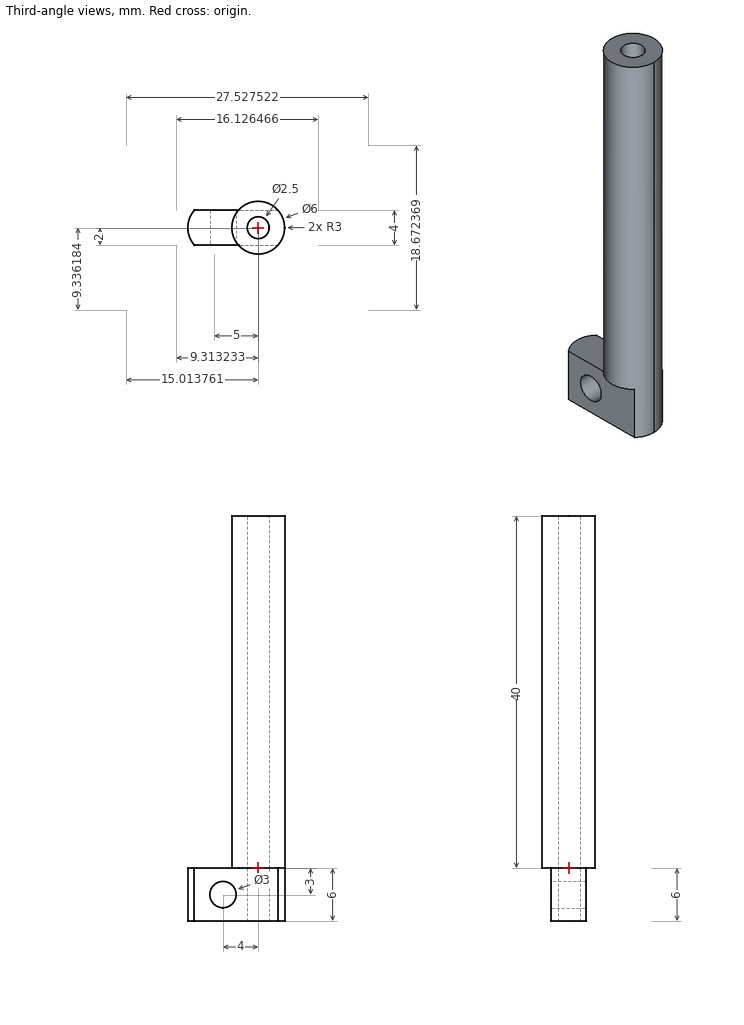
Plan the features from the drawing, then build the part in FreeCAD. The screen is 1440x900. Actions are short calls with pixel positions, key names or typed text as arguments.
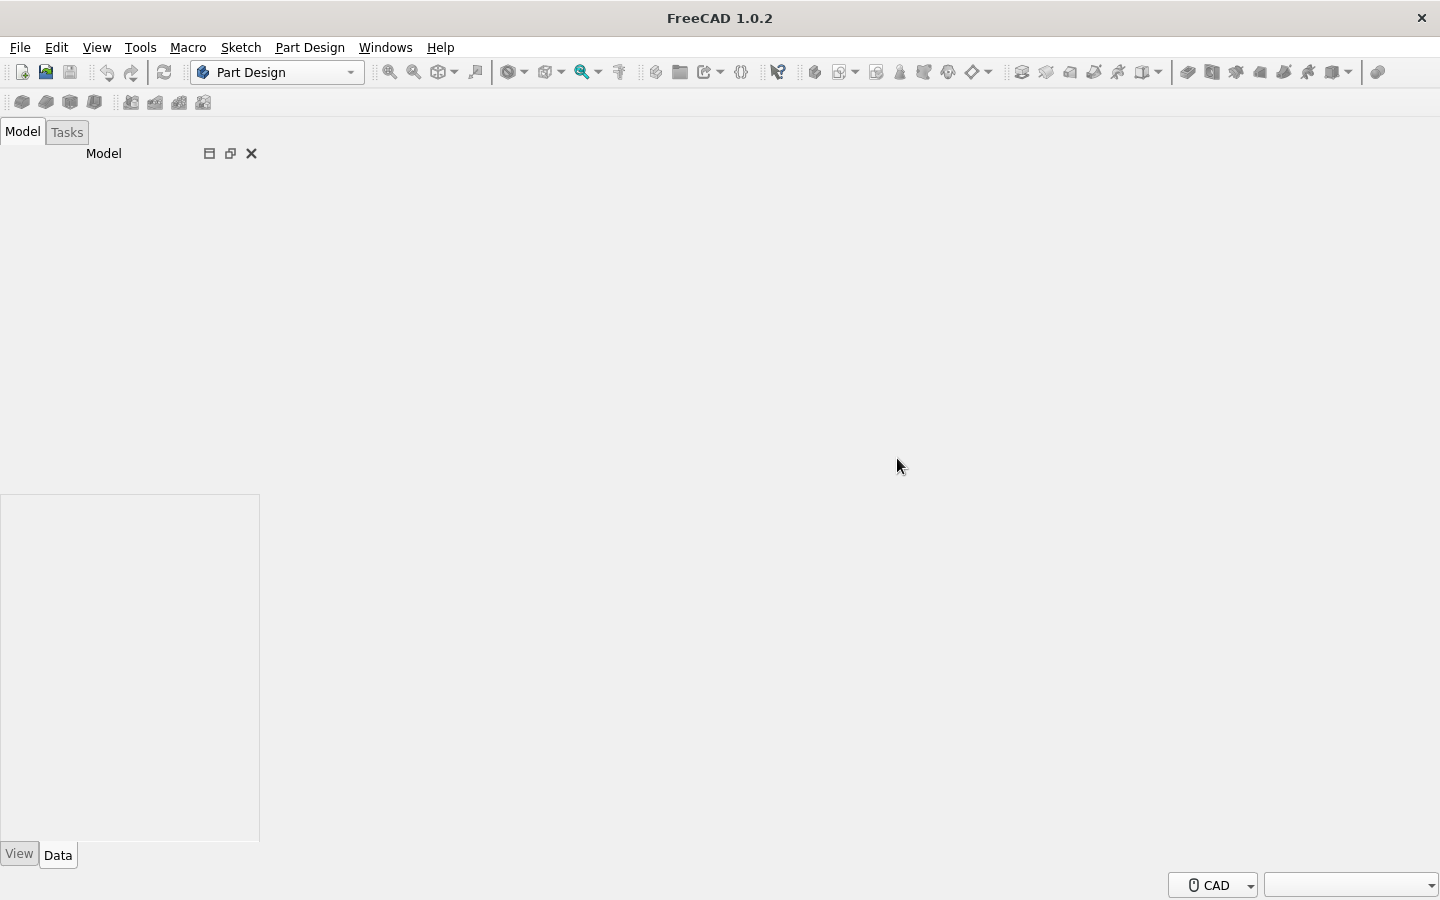
key(ctrl+n)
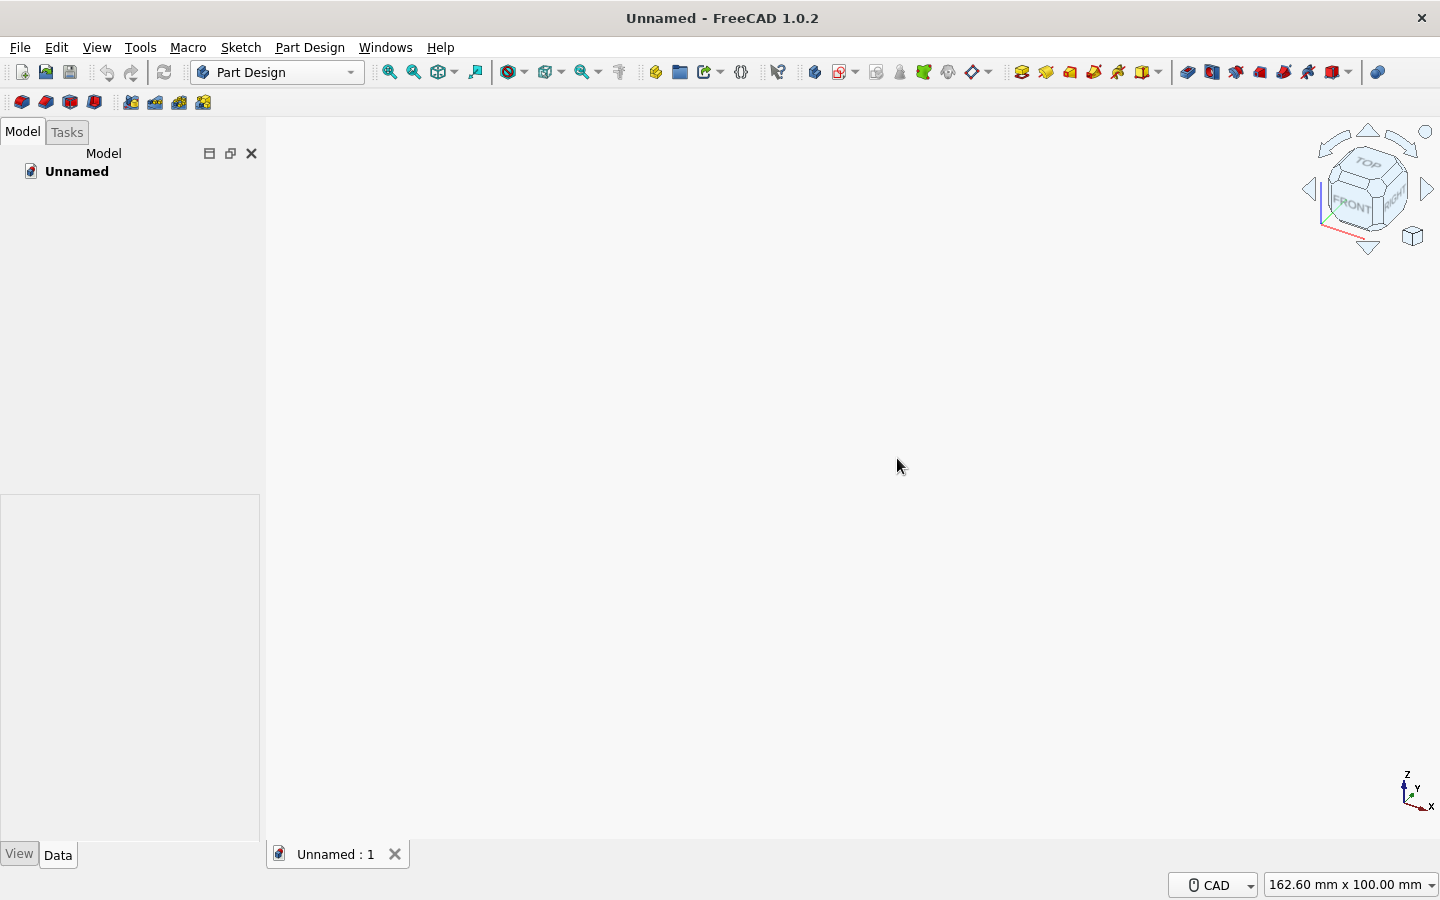
click(840, 72)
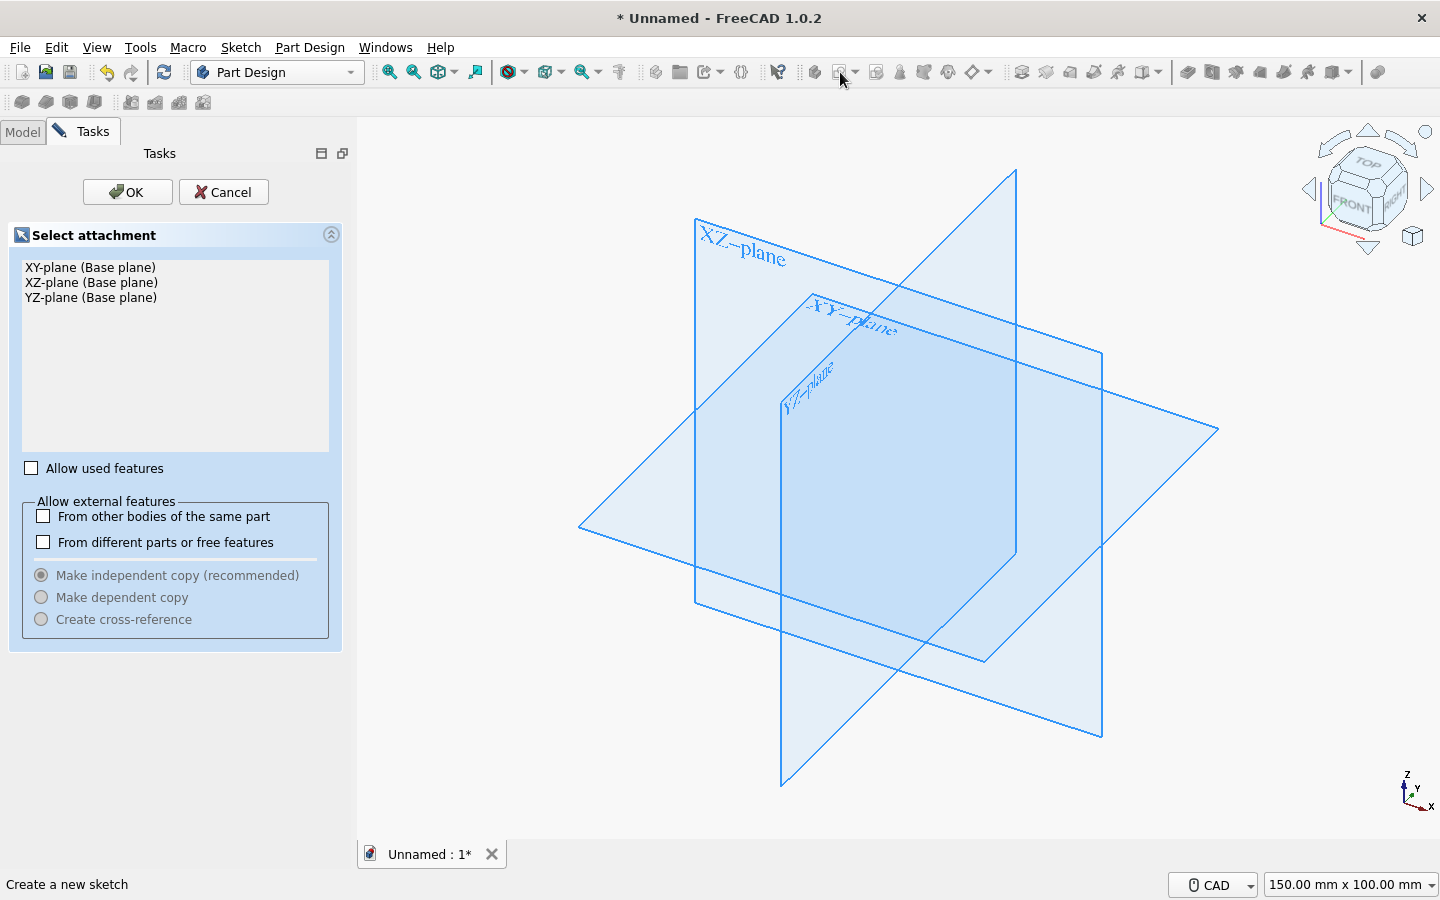
click(82, 268)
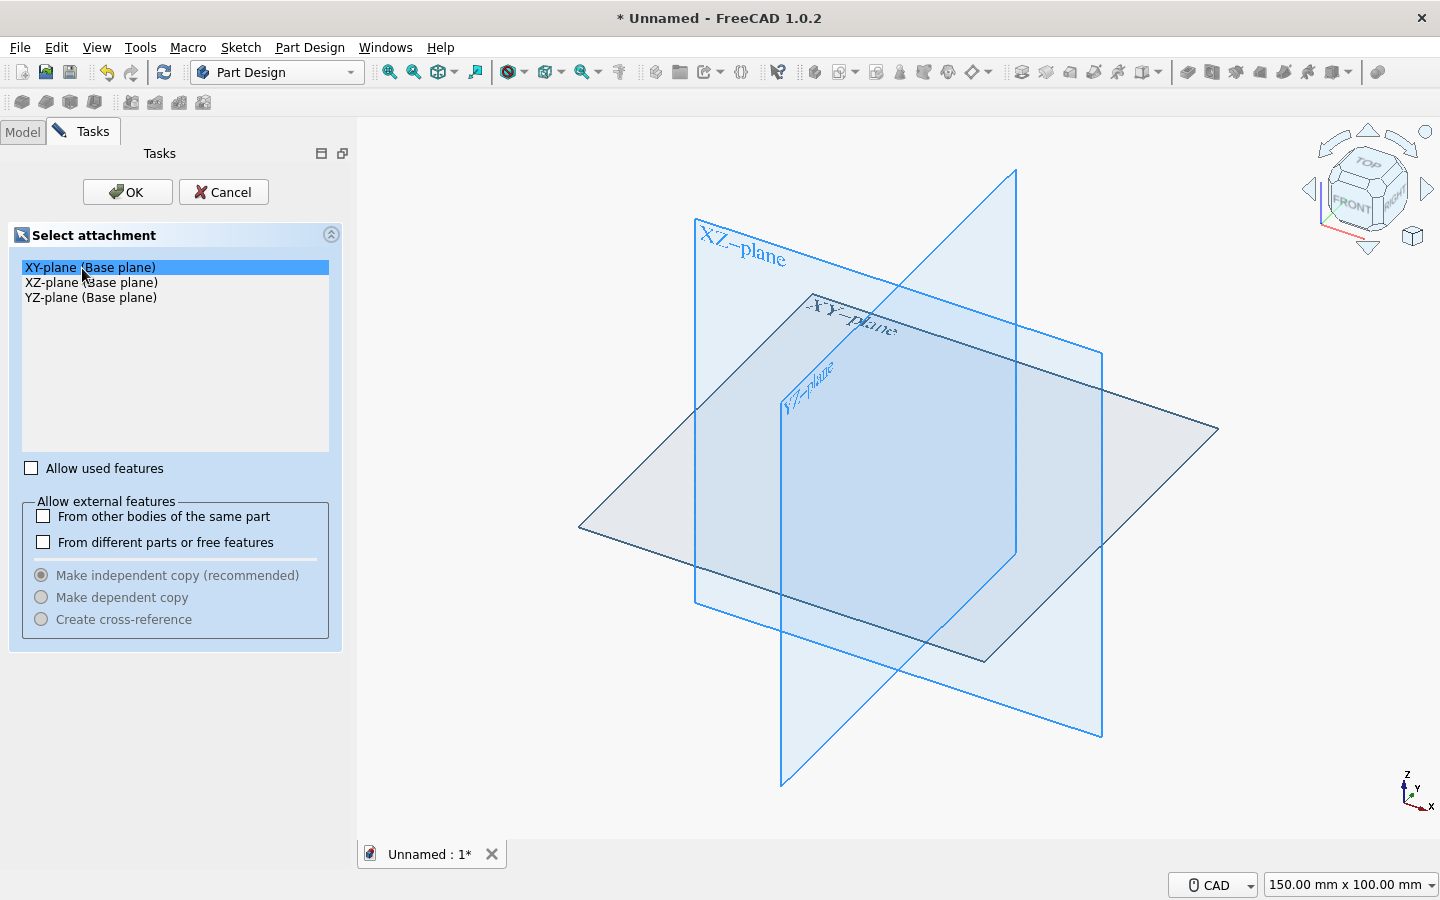
click(128, 192)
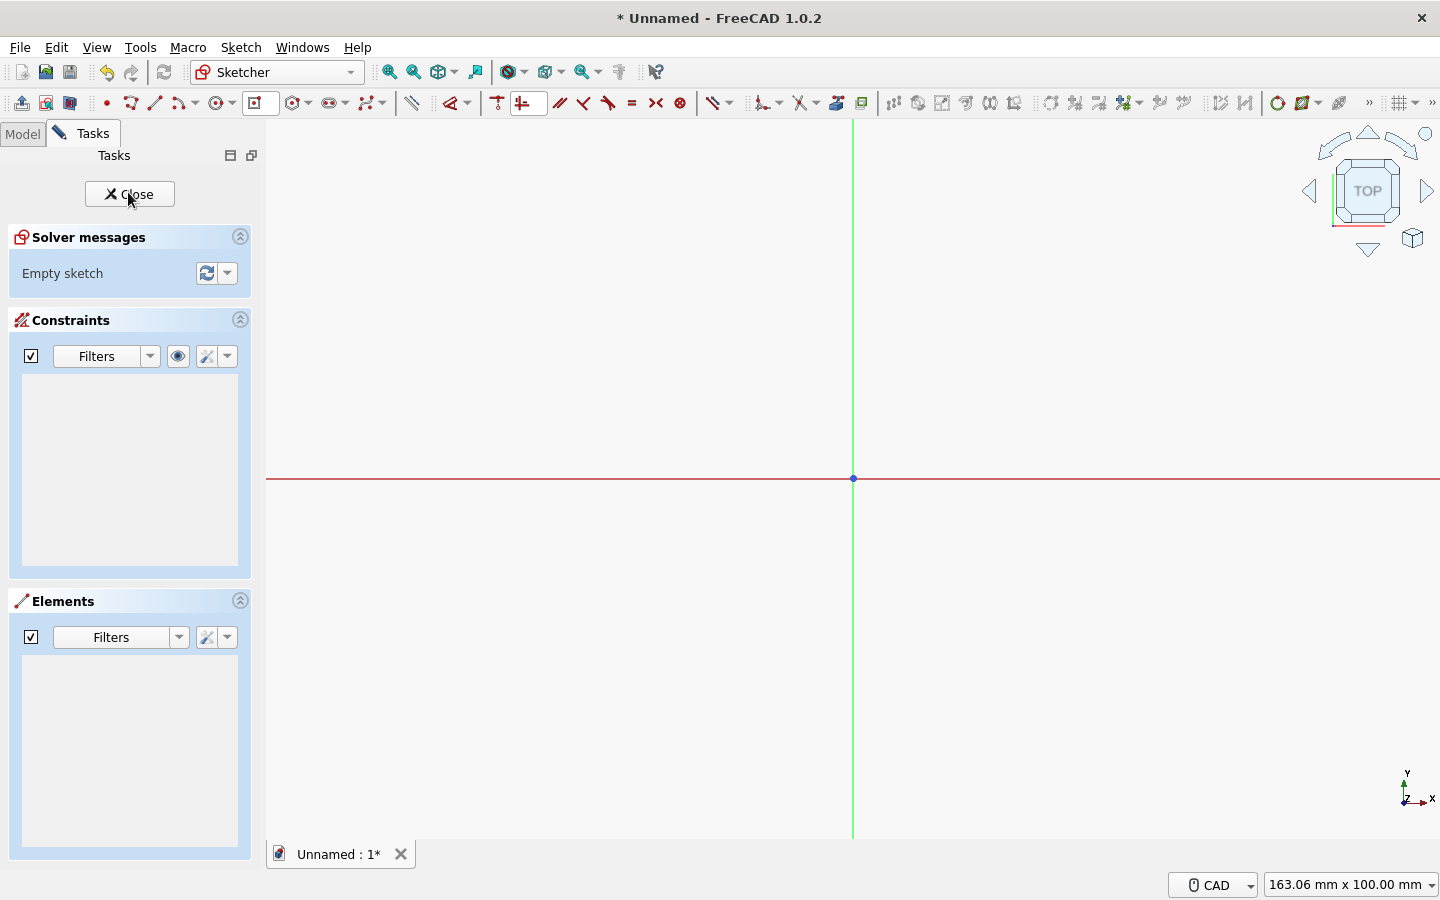
scroll(860, 479, up, 12)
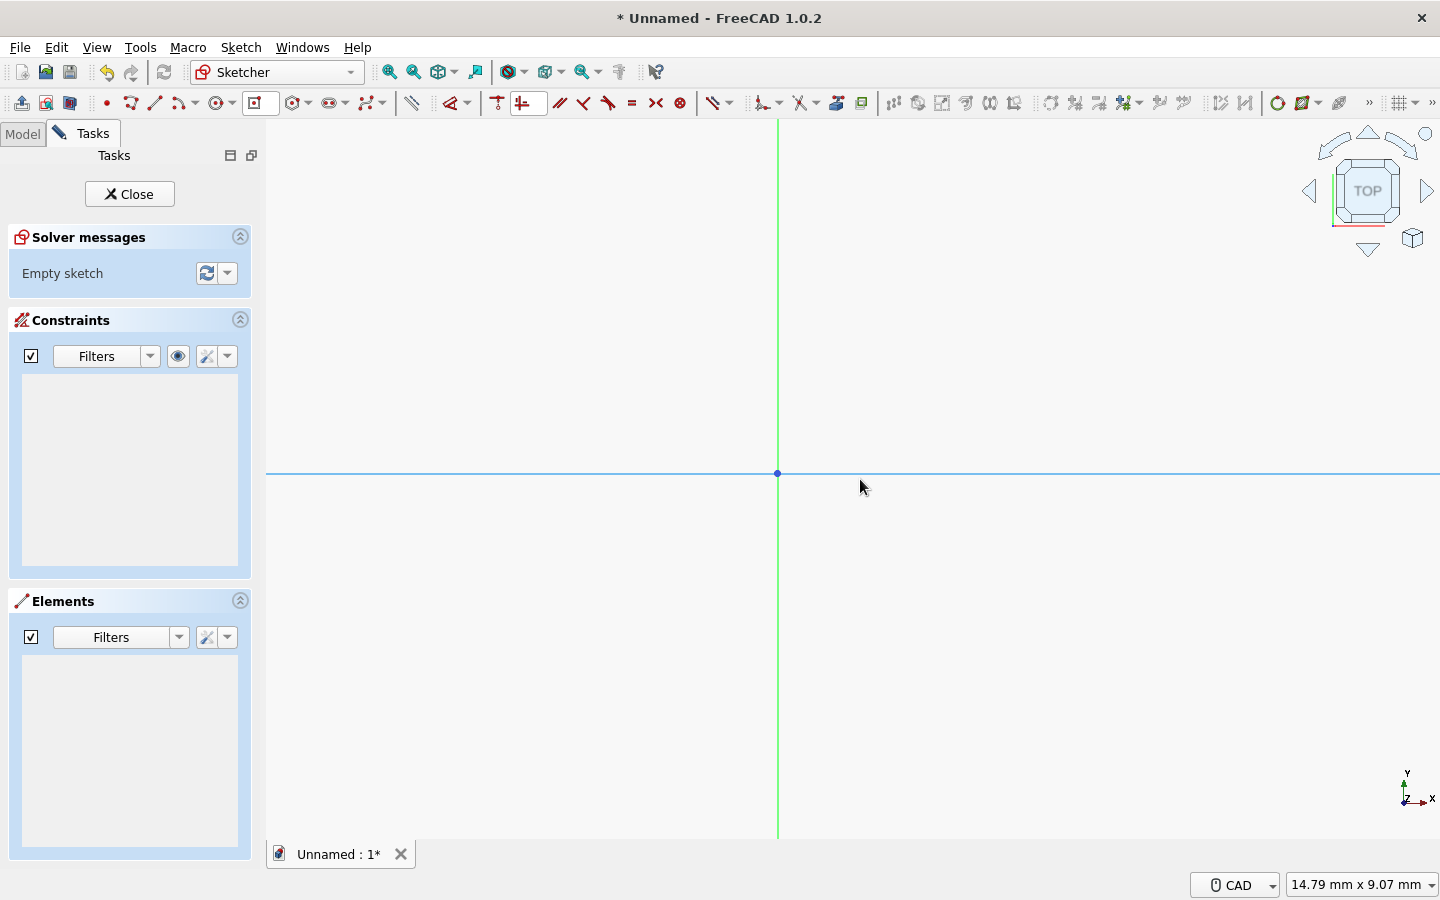
key(g)
key(c)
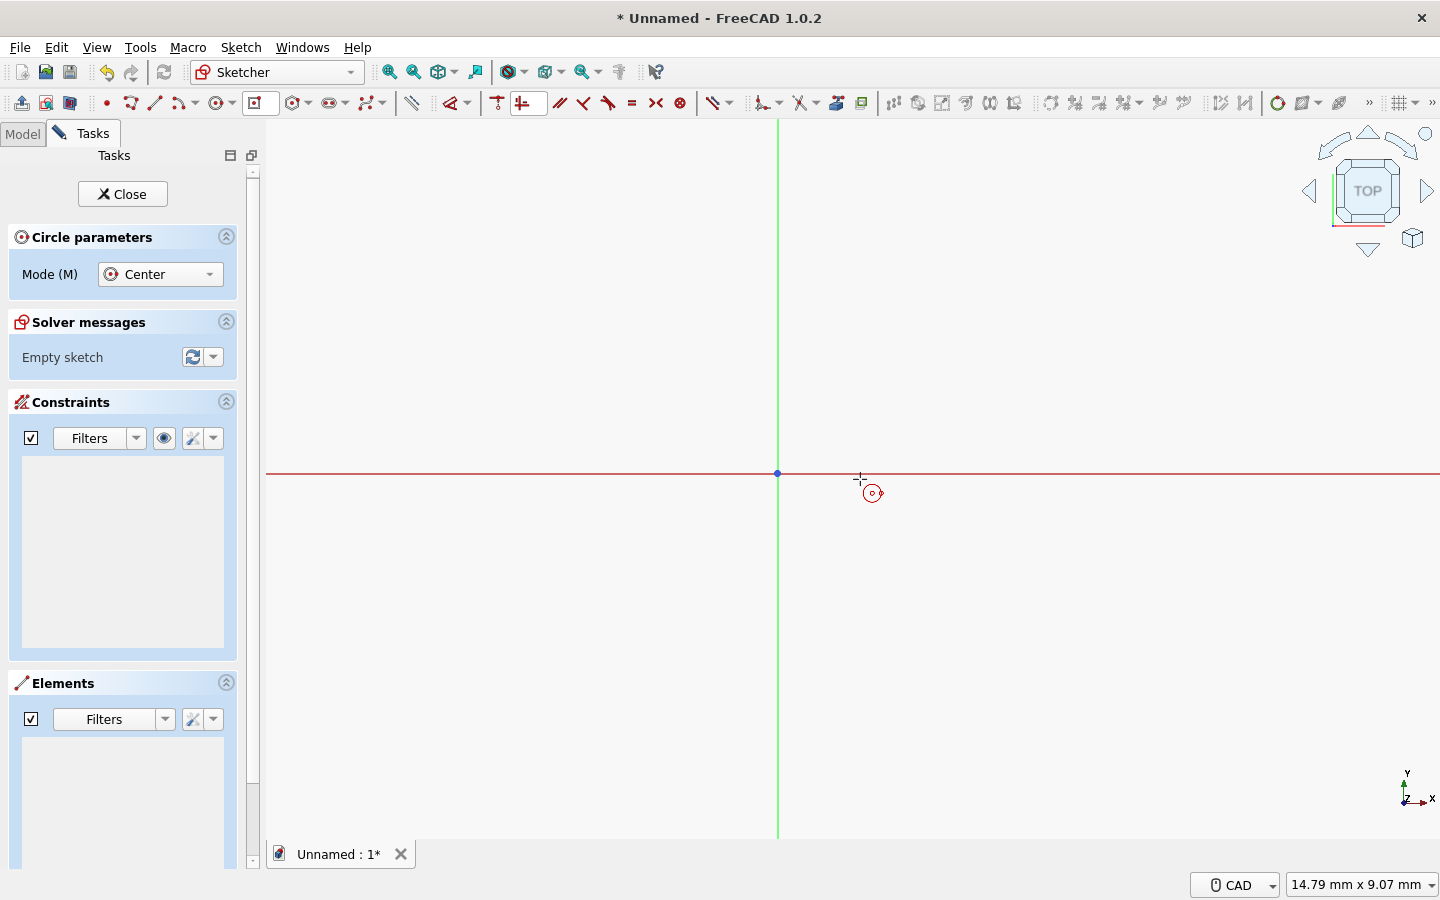
click(778, 474)
move(946, 306)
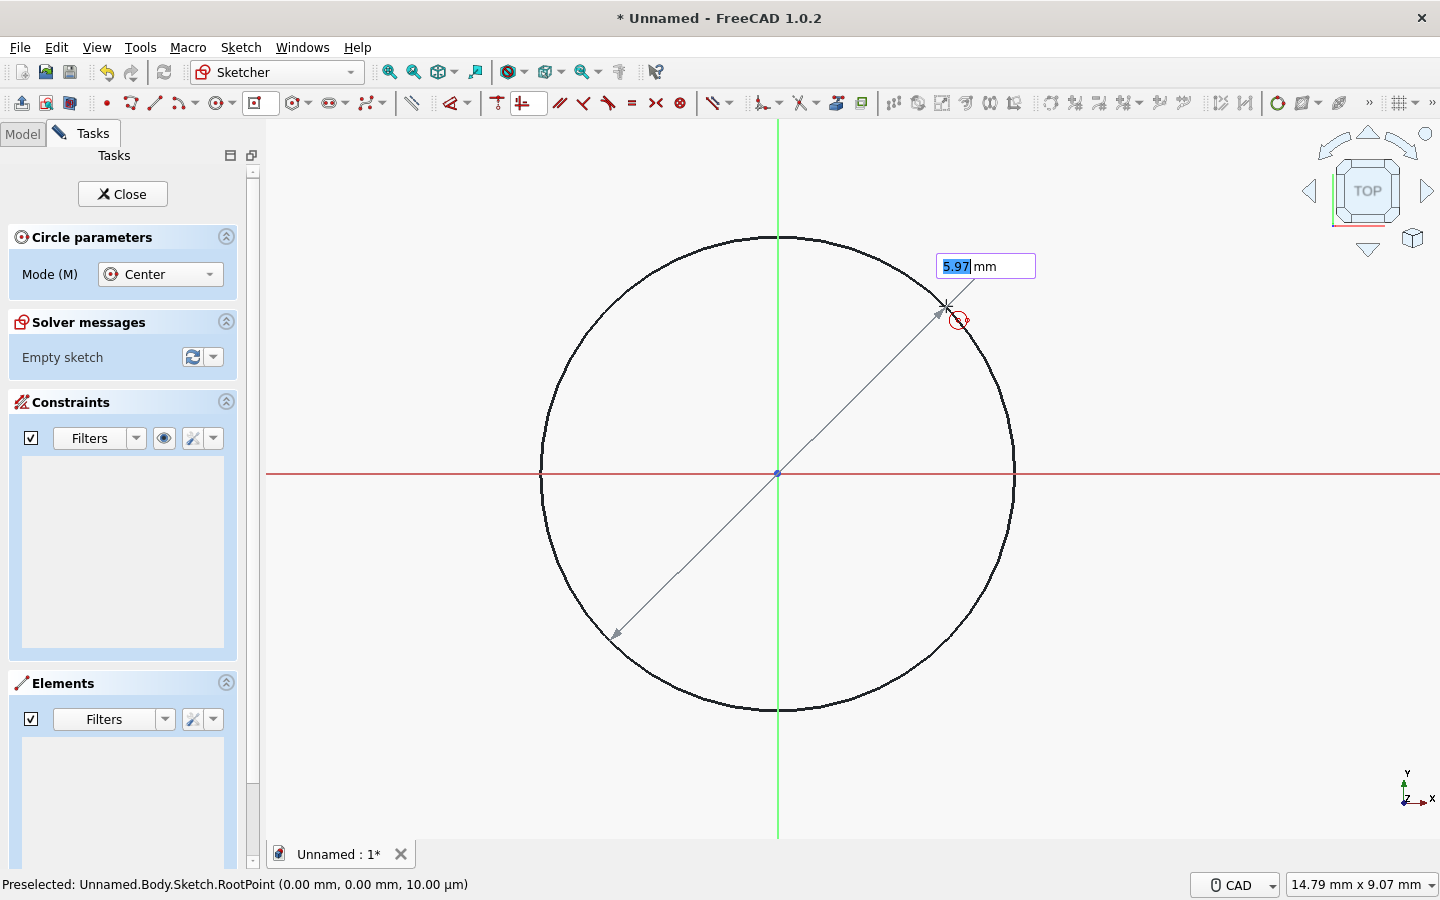
text(6)
key(Return)